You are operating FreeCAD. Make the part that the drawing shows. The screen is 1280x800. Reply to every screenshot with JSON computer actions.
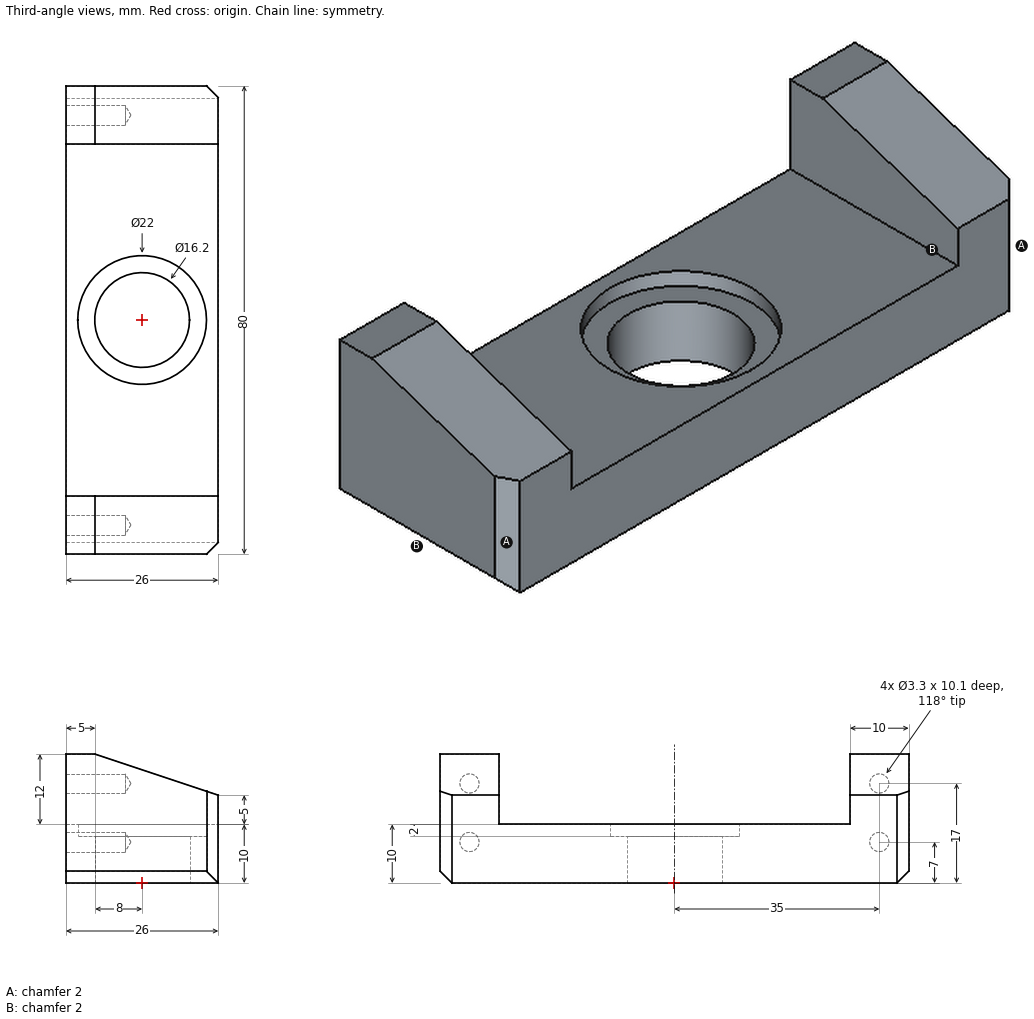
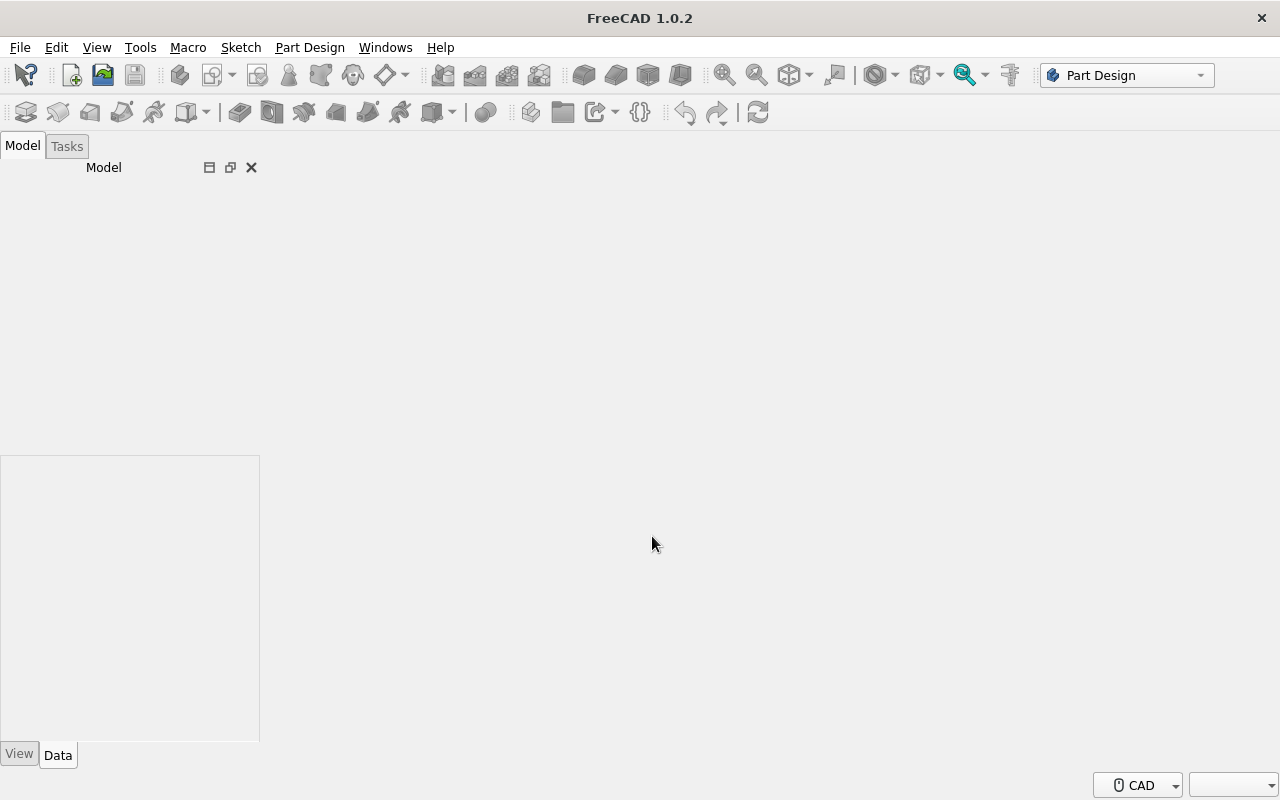
{"action": "left_click", "coordinate": [72, 76]}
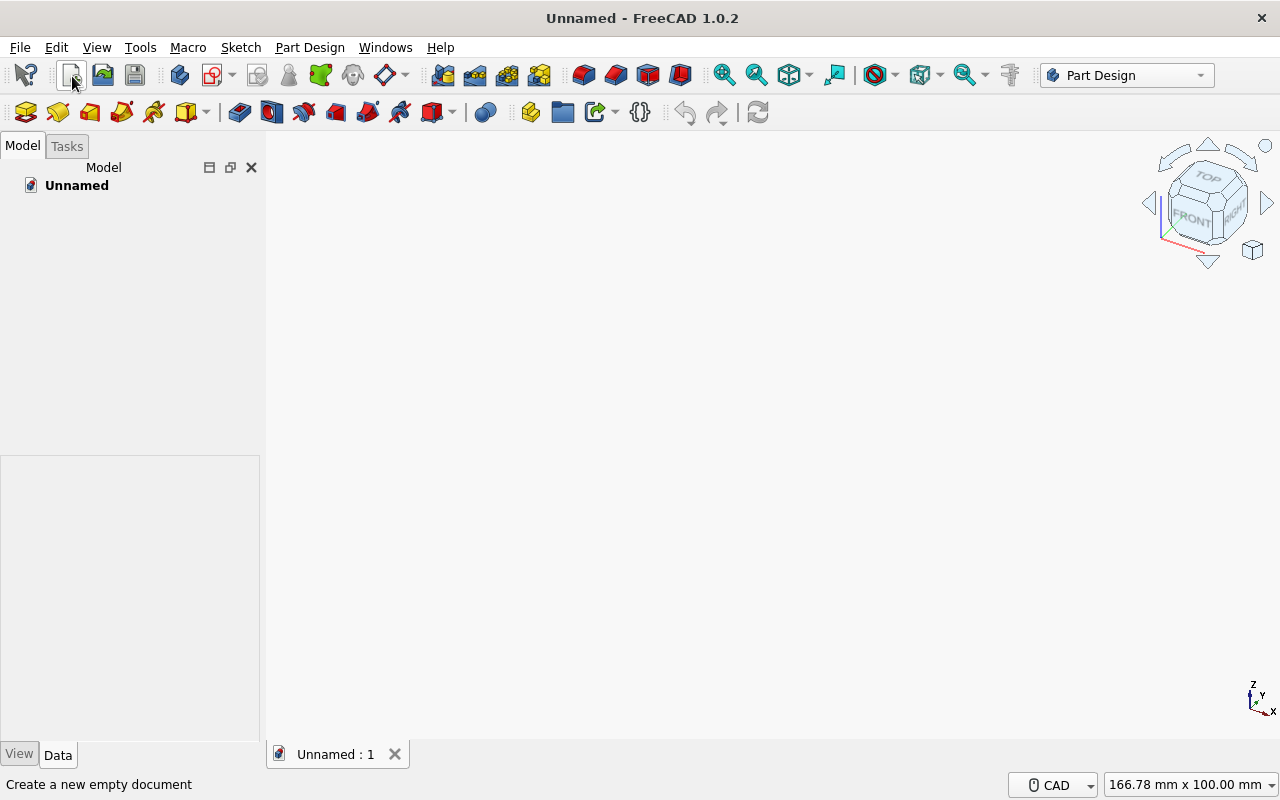
{"action": "left_click", "coordinate": [212, 76]}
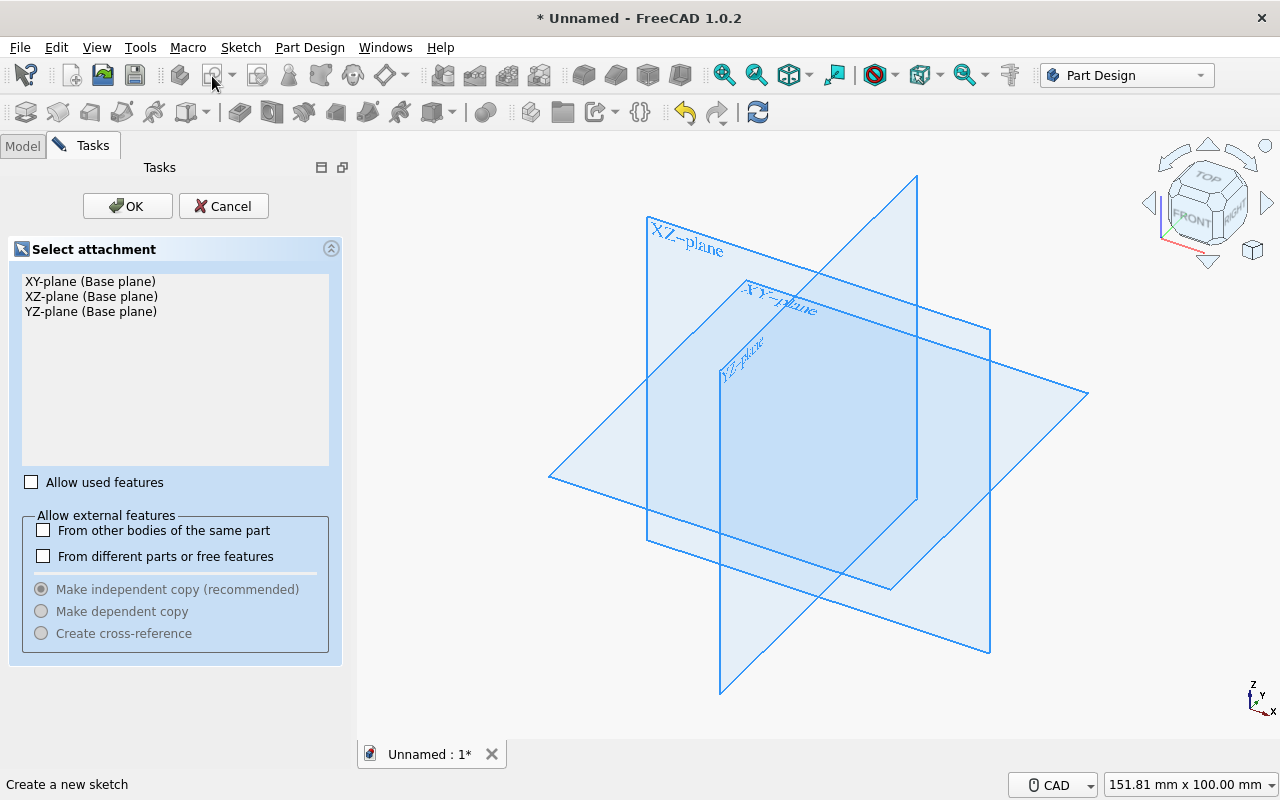
{"action": "left_click", "coordinate": [82, 282]}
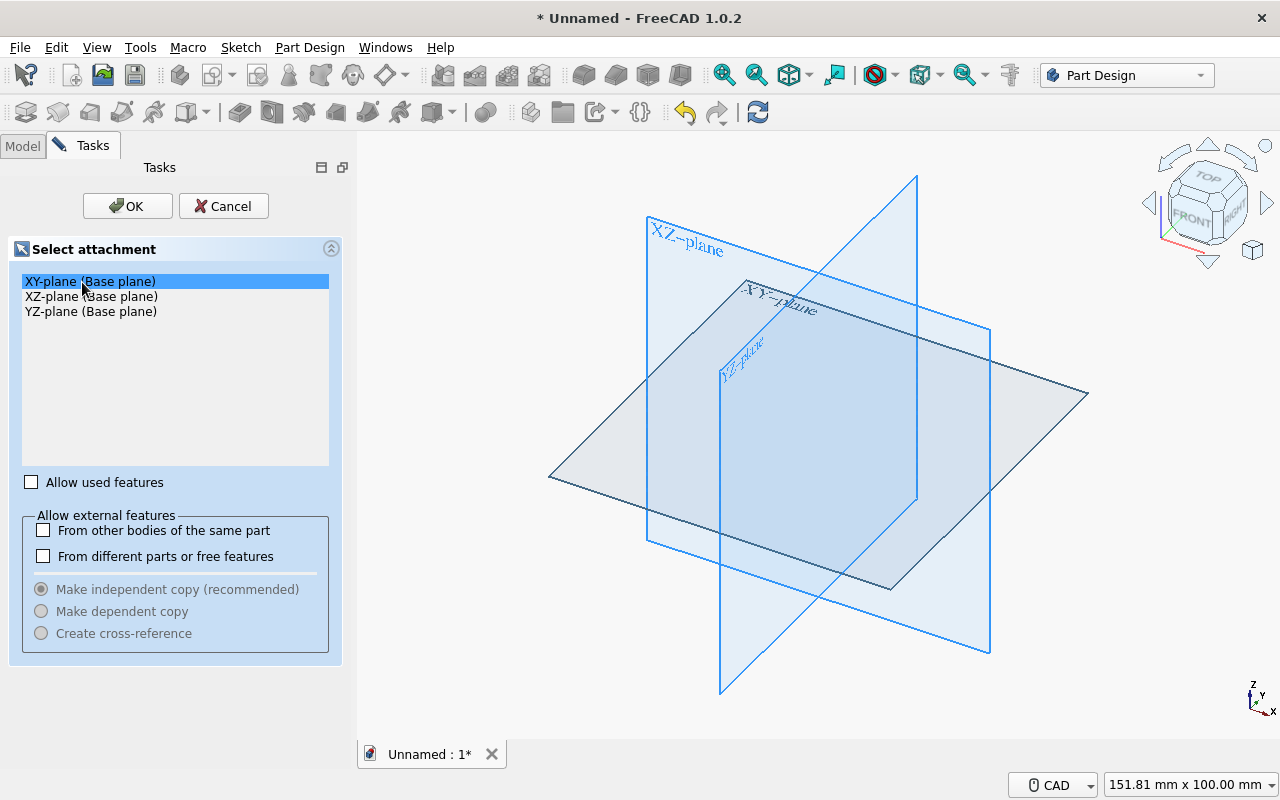
{"action": "left_click", "coordinate": [128, 206]}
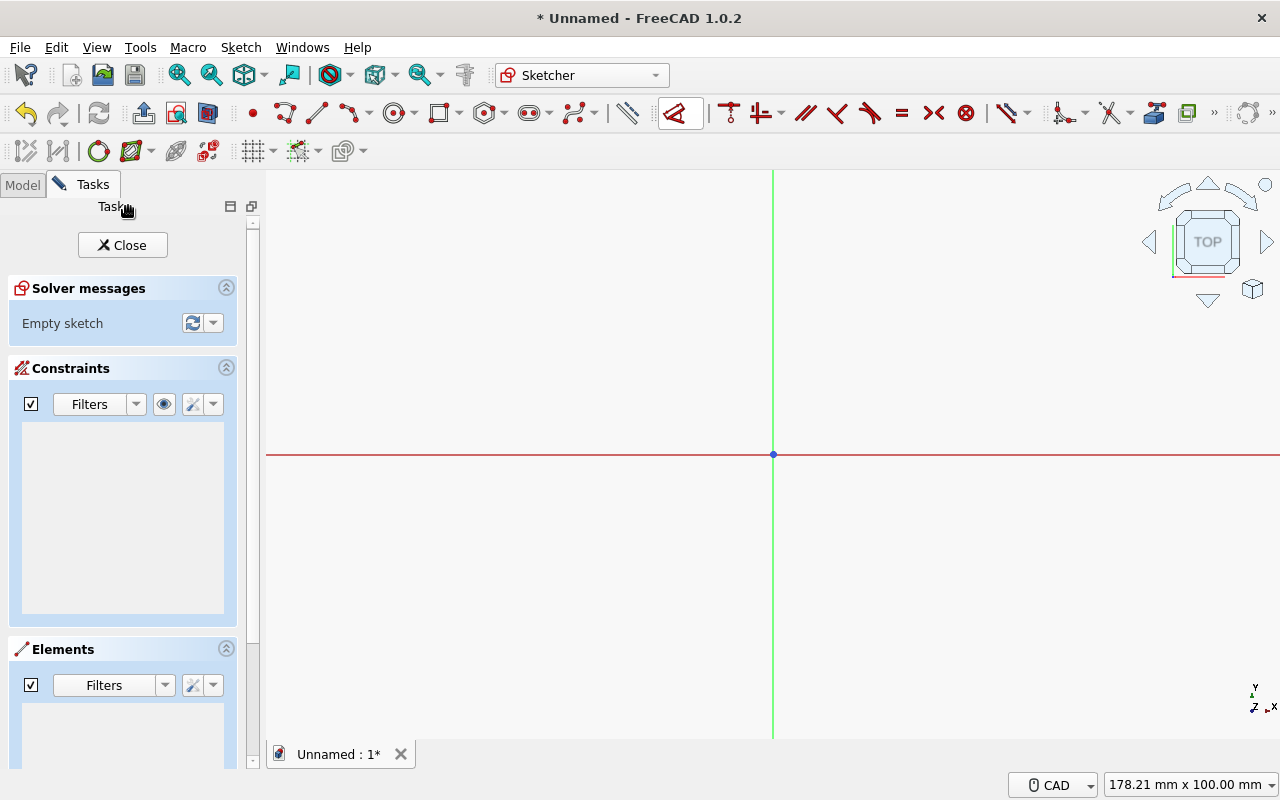
{"action": "key", "text": "g v"}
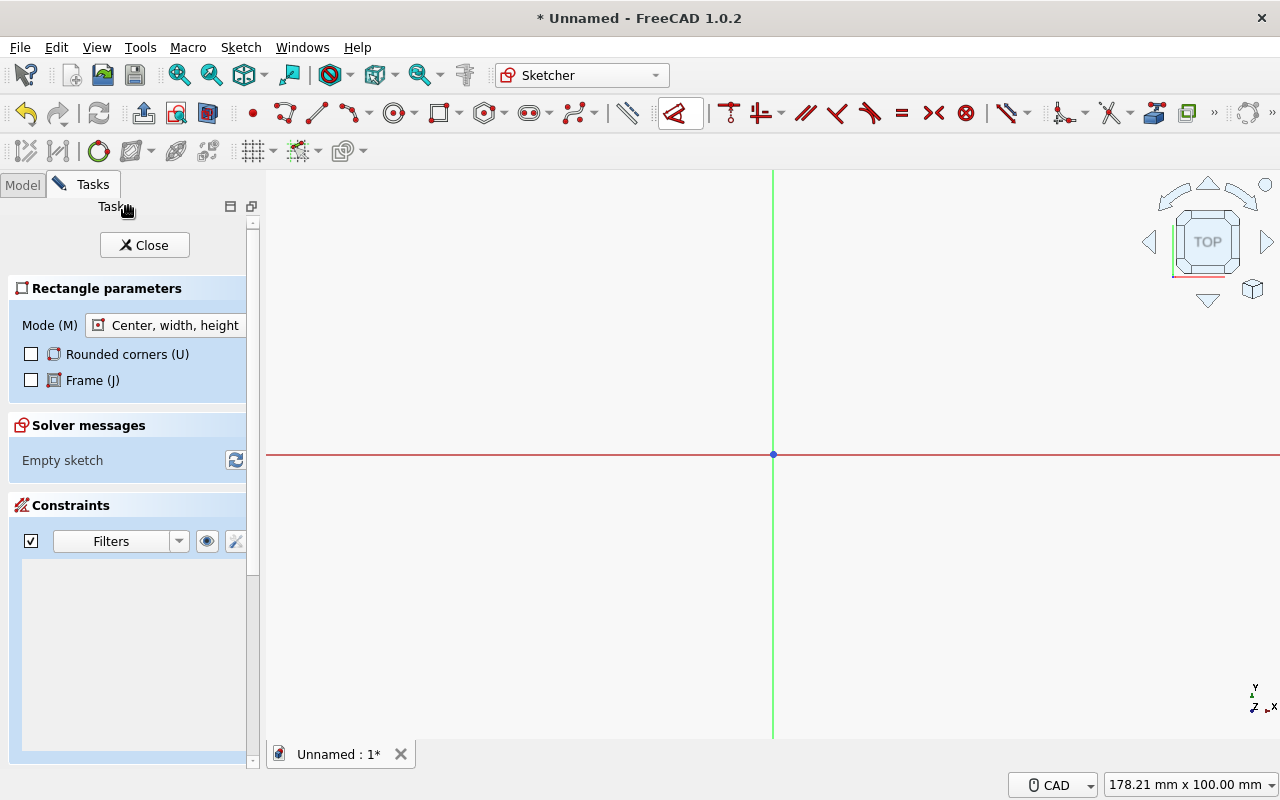
{"action": "left_click", "coordinate": [773, 454]}
{"action": "left_click", "coordinate": [847, 227]}
{"action": "key", "text": "Escape"}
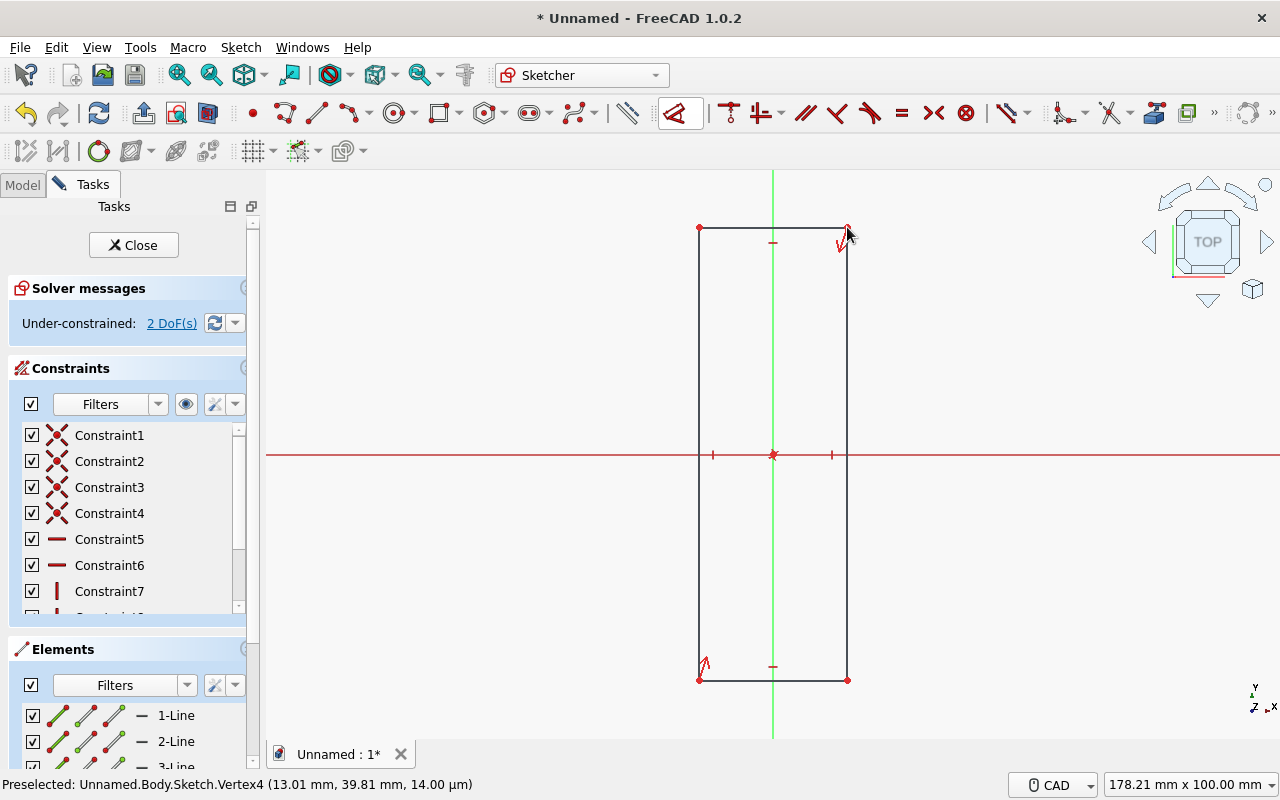
{"action": "left_click", "coordinate": [743, 681]}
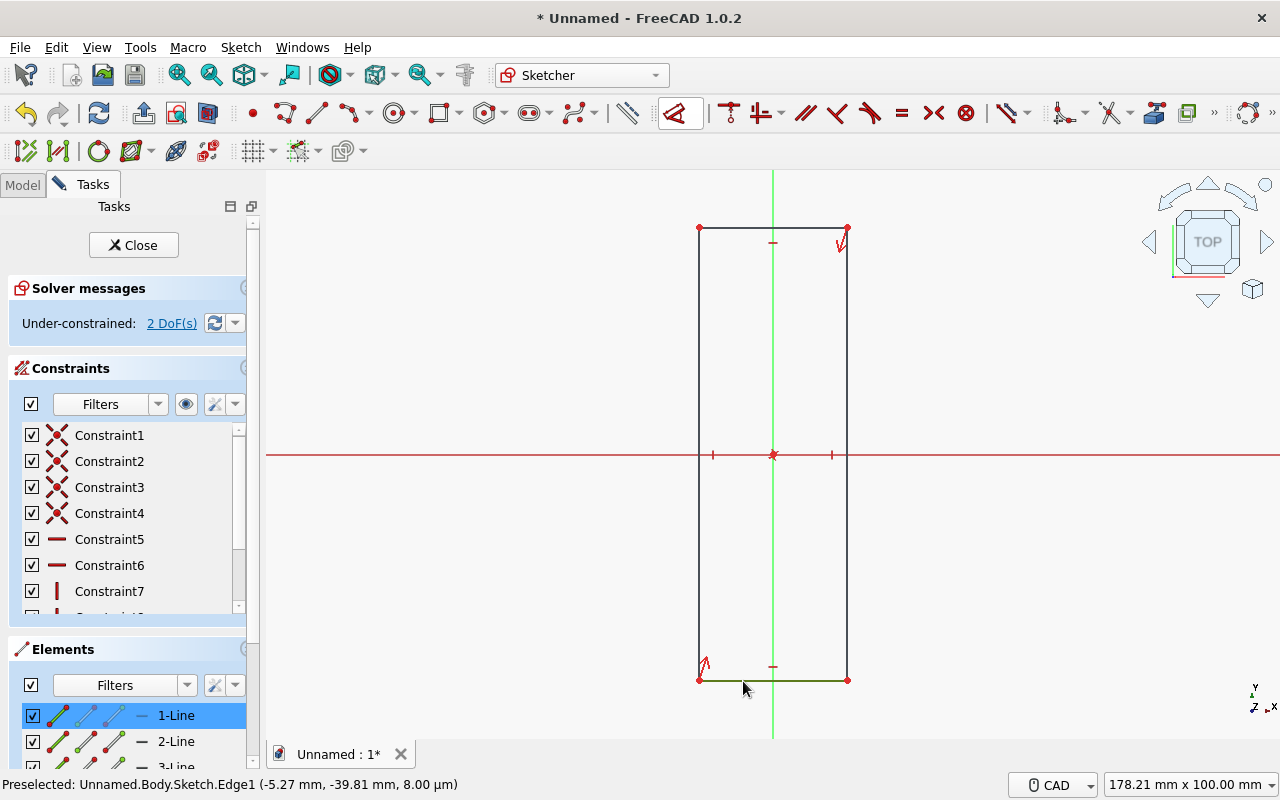
{"action": "left_click", "coordinate": [698, 114]}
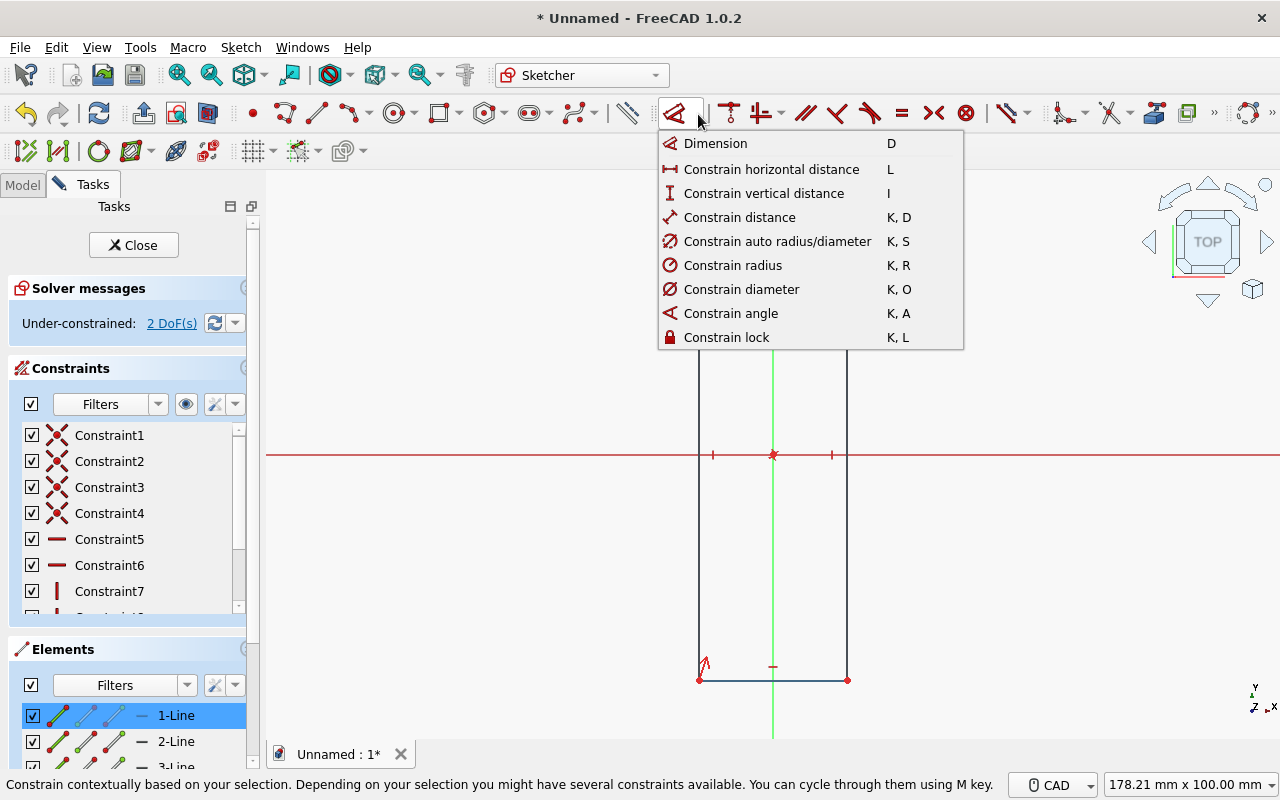
{"action": "left_click", "coordinate": [811, 169]}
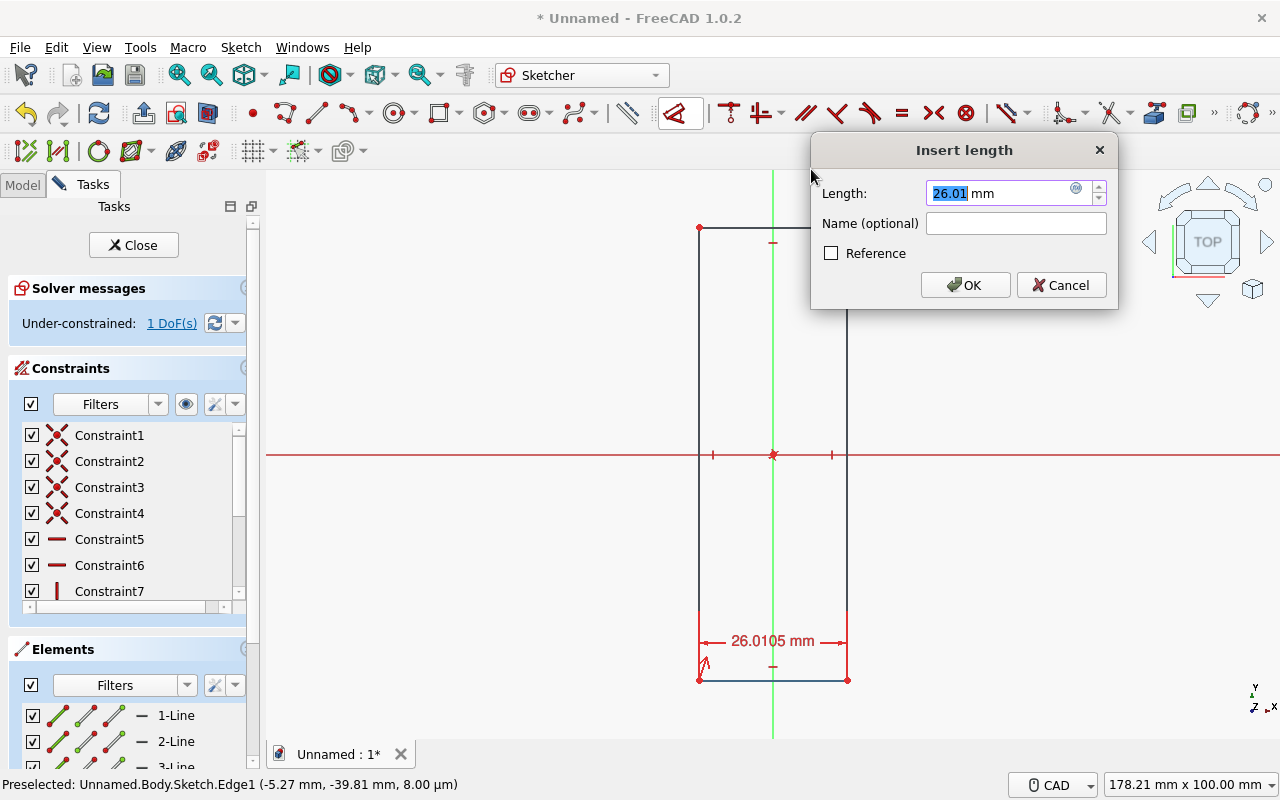
{"action": "type", "text": "26"}
{"action": "key", "text": "Return"}